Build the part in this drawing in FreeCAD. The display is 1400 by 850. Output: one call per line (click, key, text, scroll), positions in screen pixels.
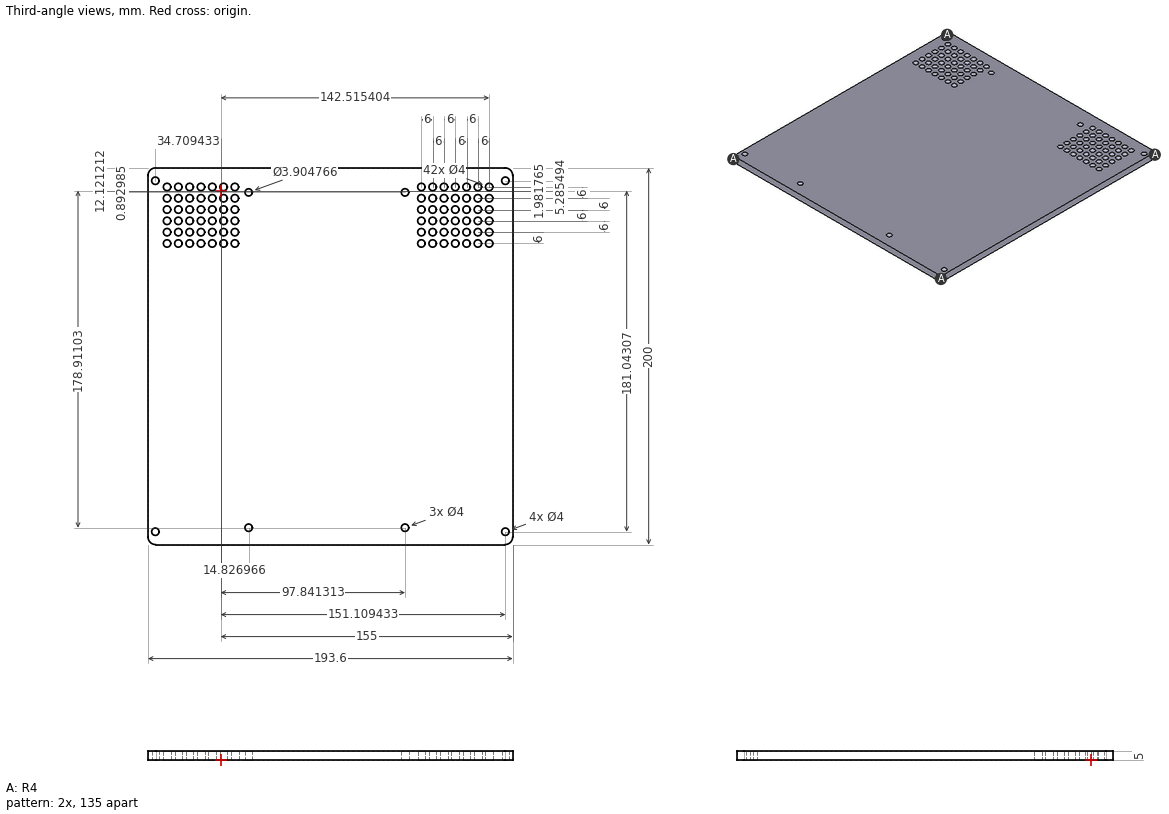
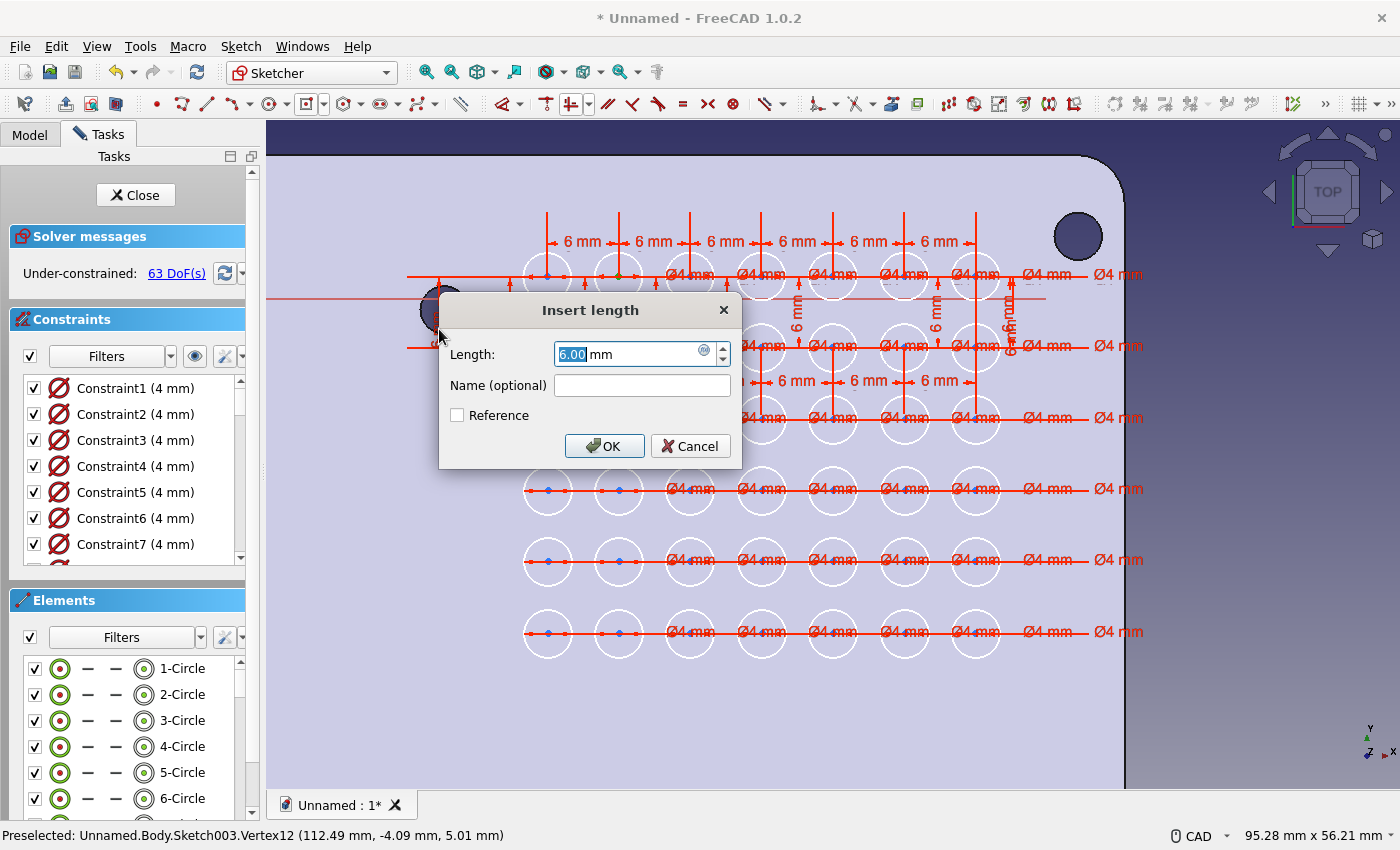
text(6)
key(Return)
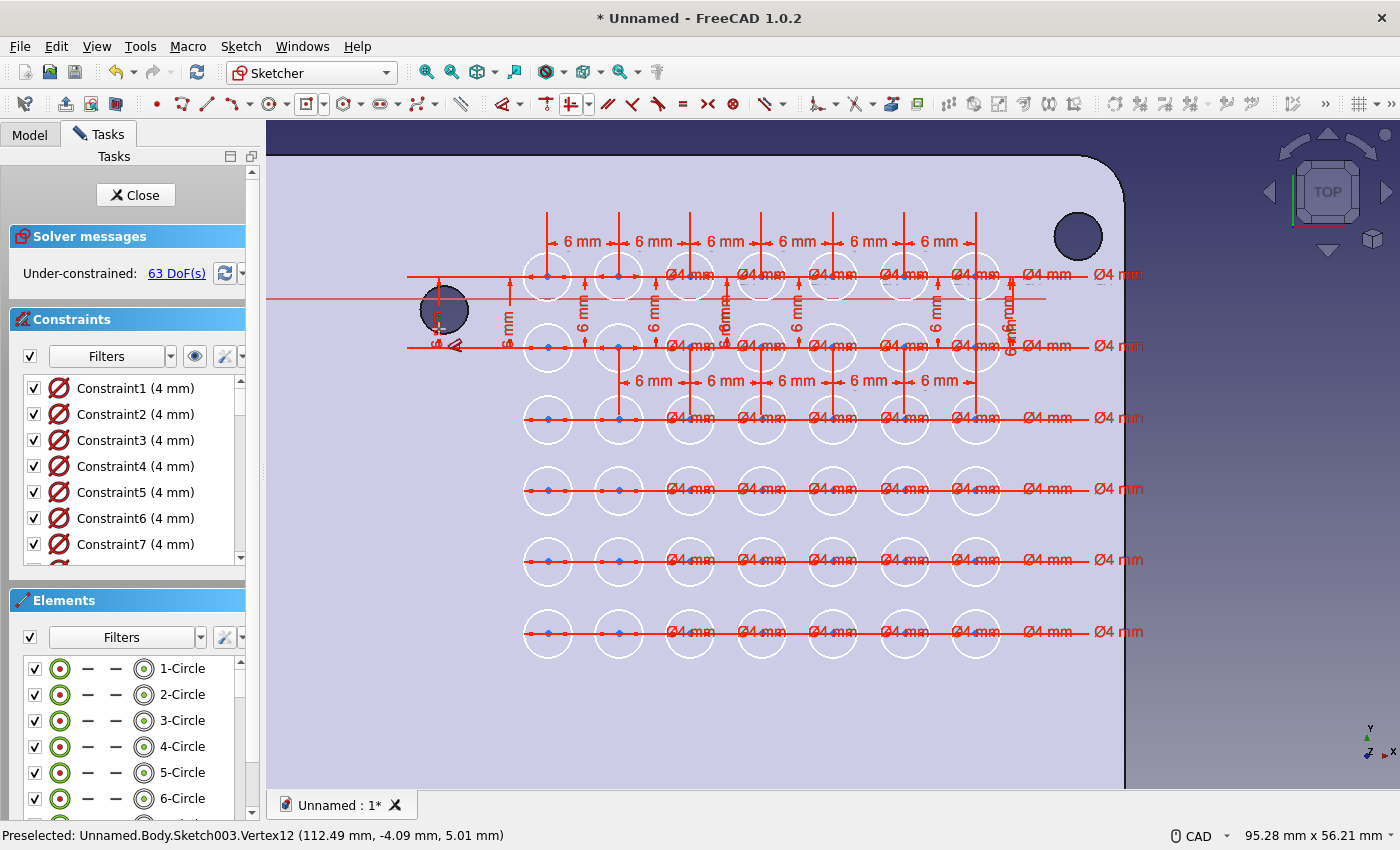
click(547, 277)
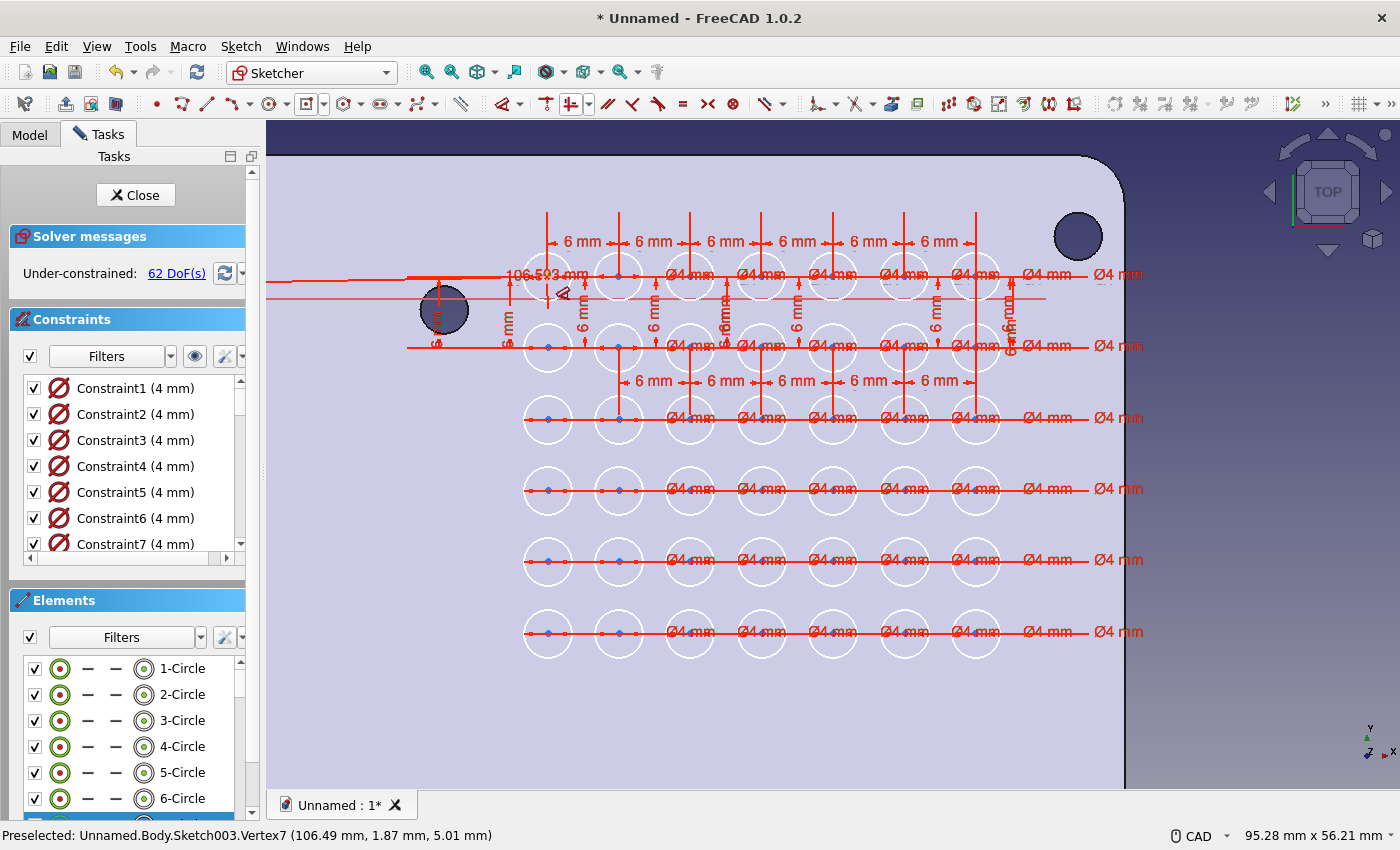
click(619, 348)
click(367, 313)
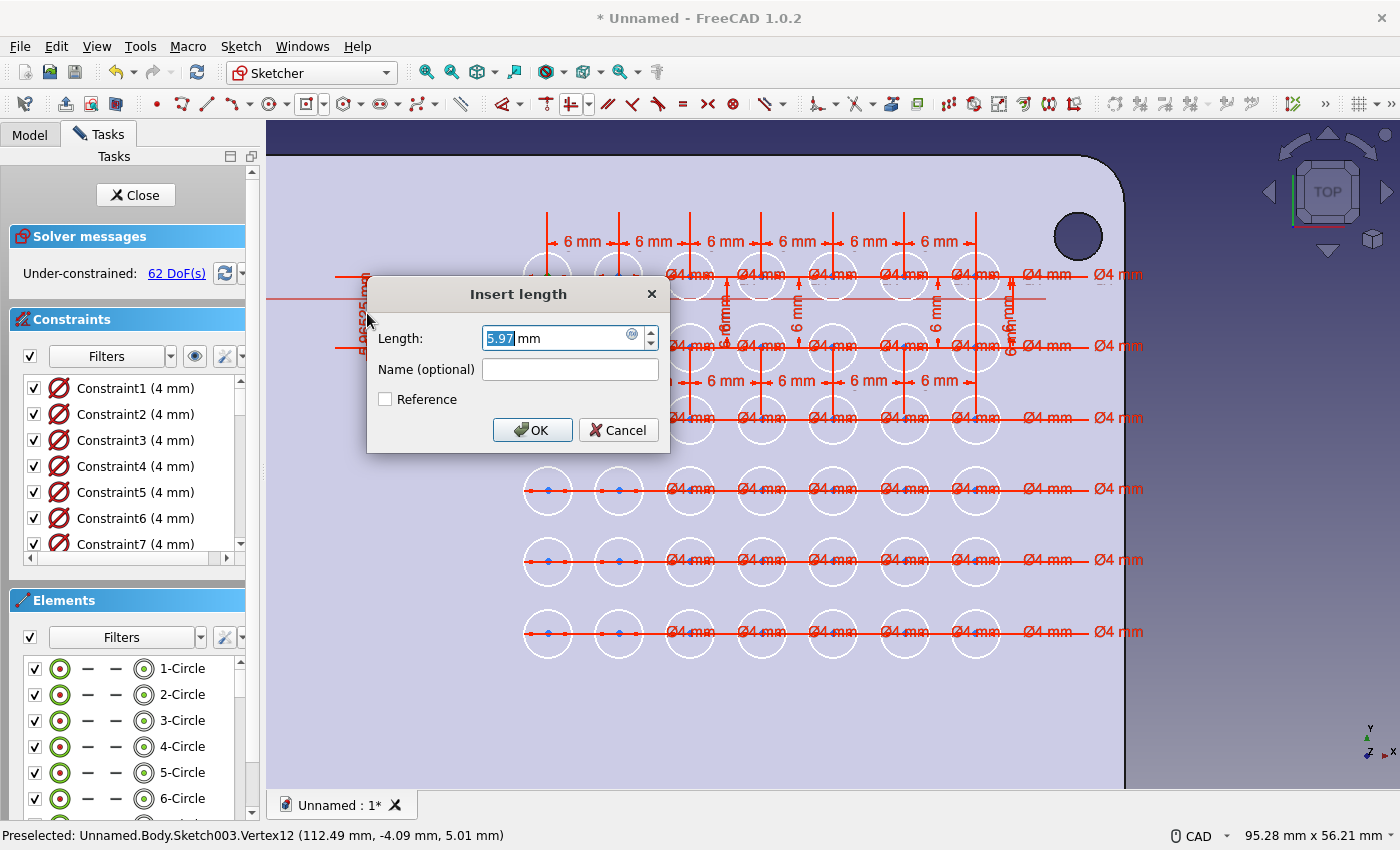
text(6)
key(Return)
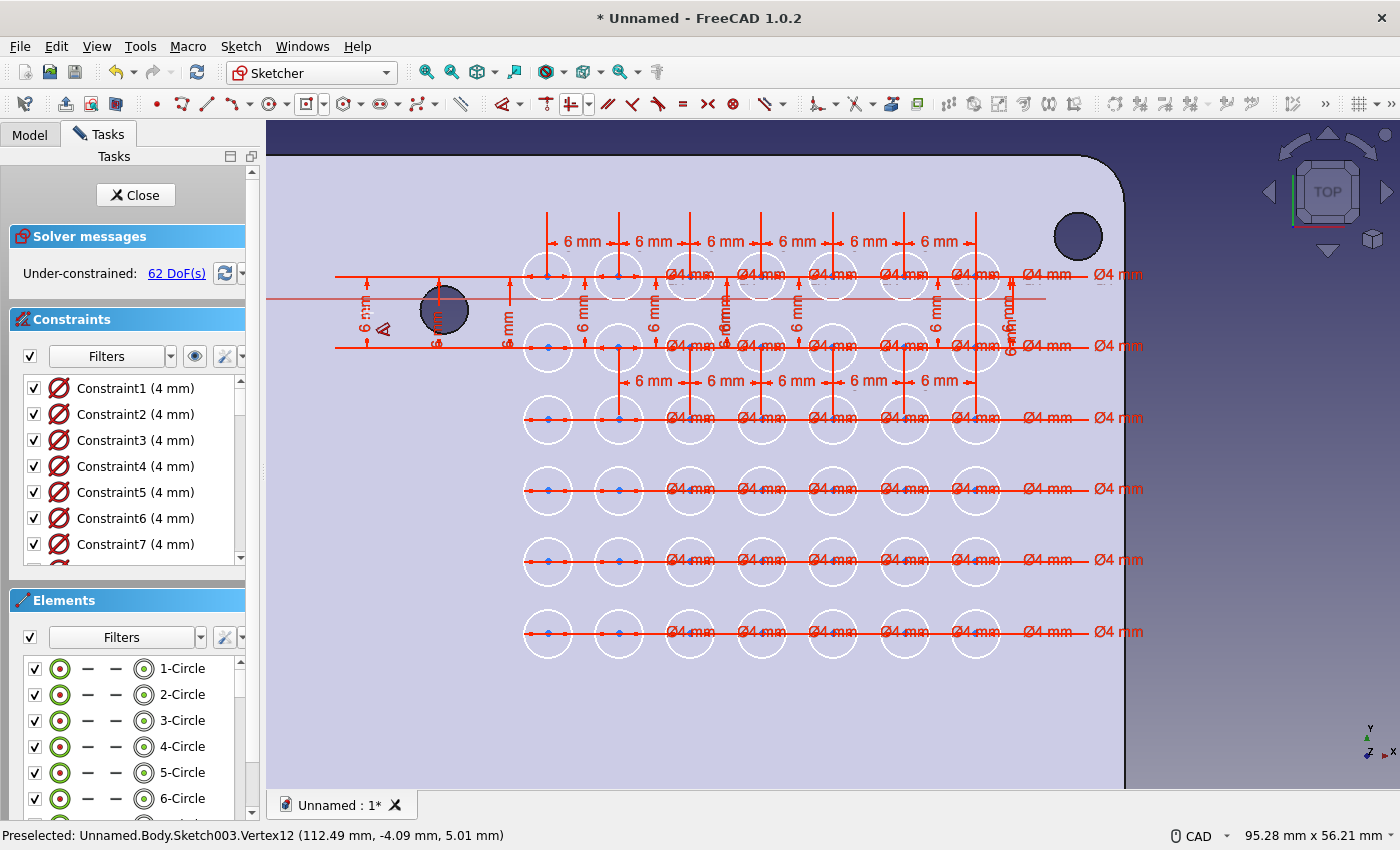
click(619, 348)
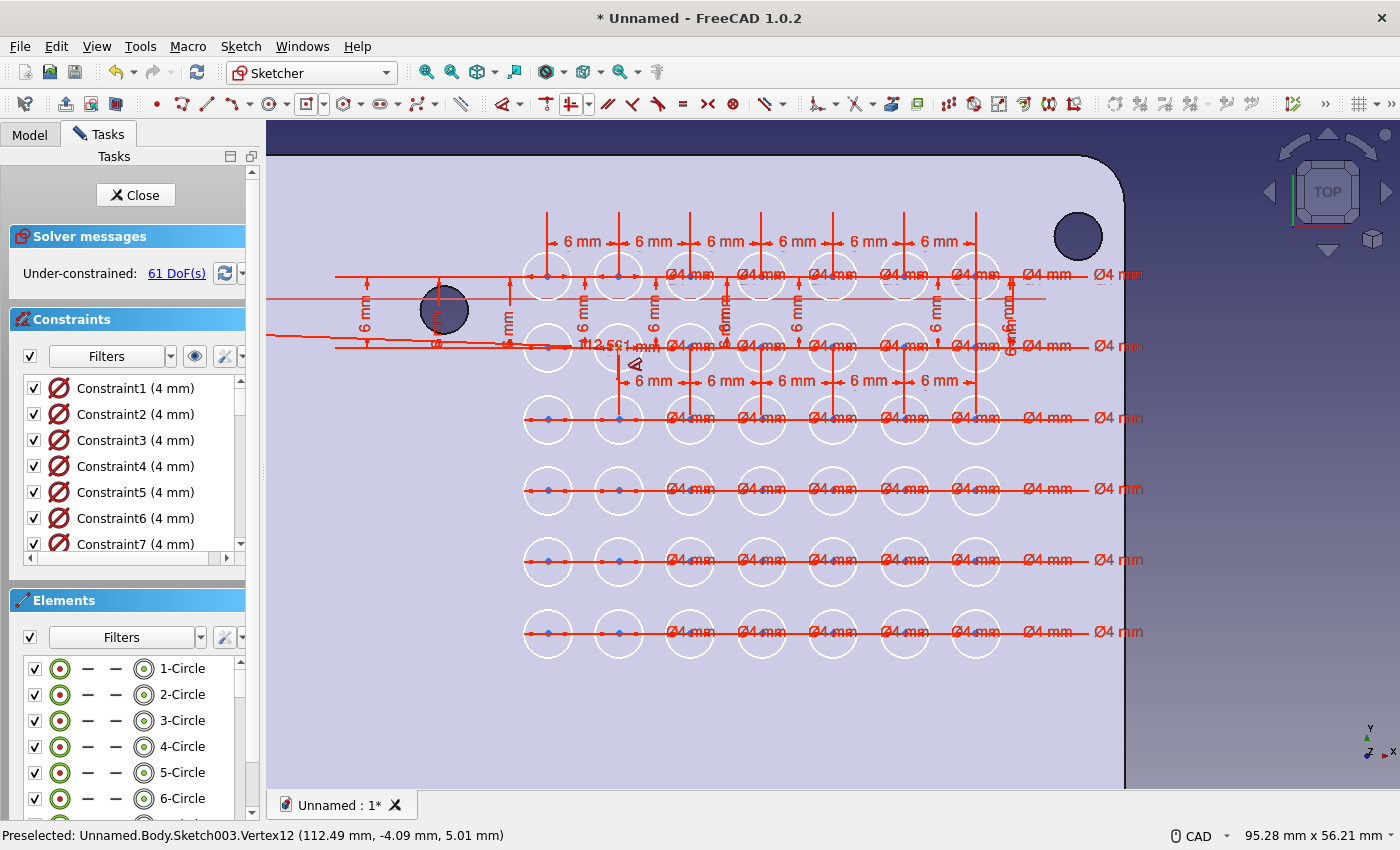
click(548, 348)
click(583, 382)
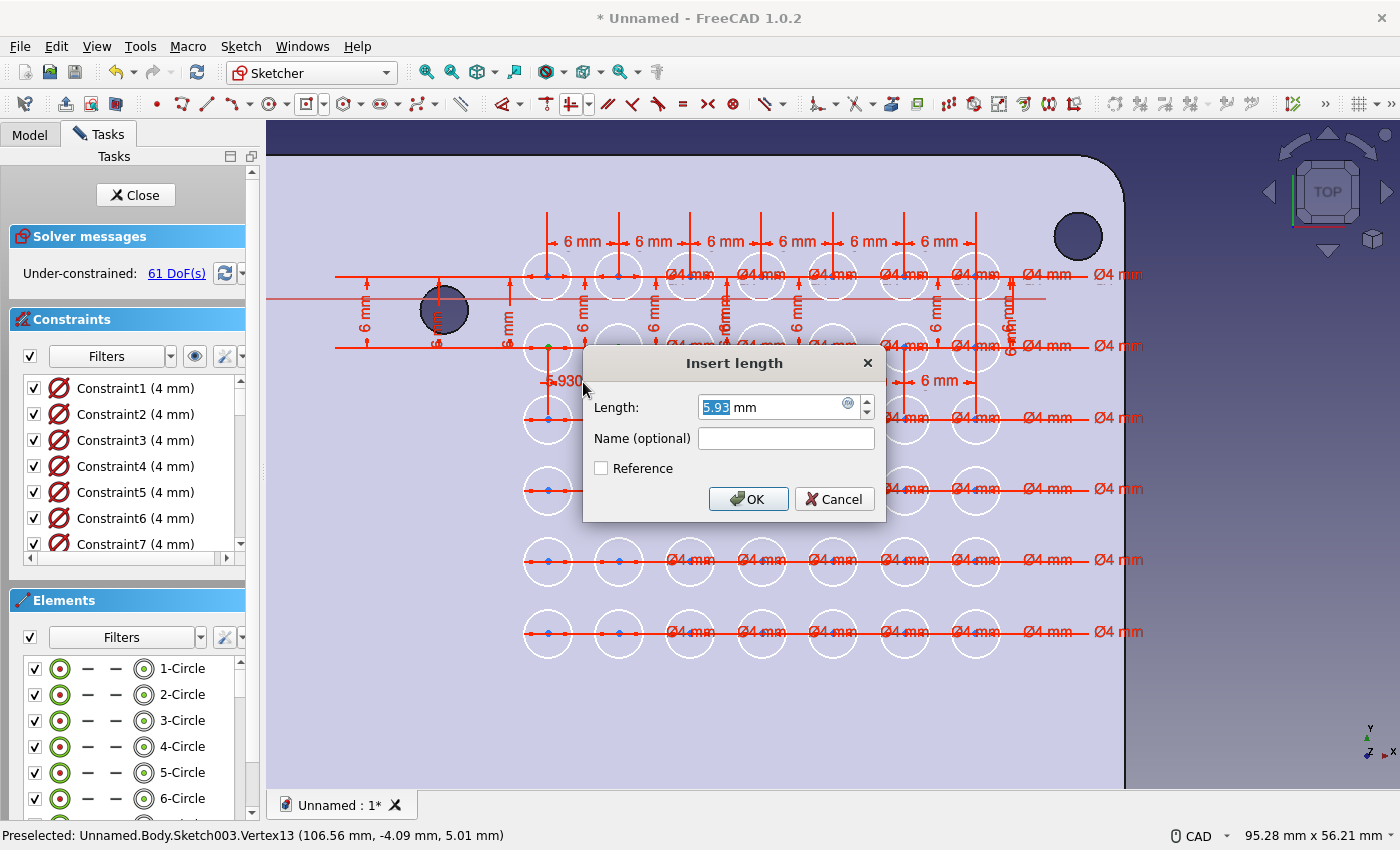
text(6)
key(Return)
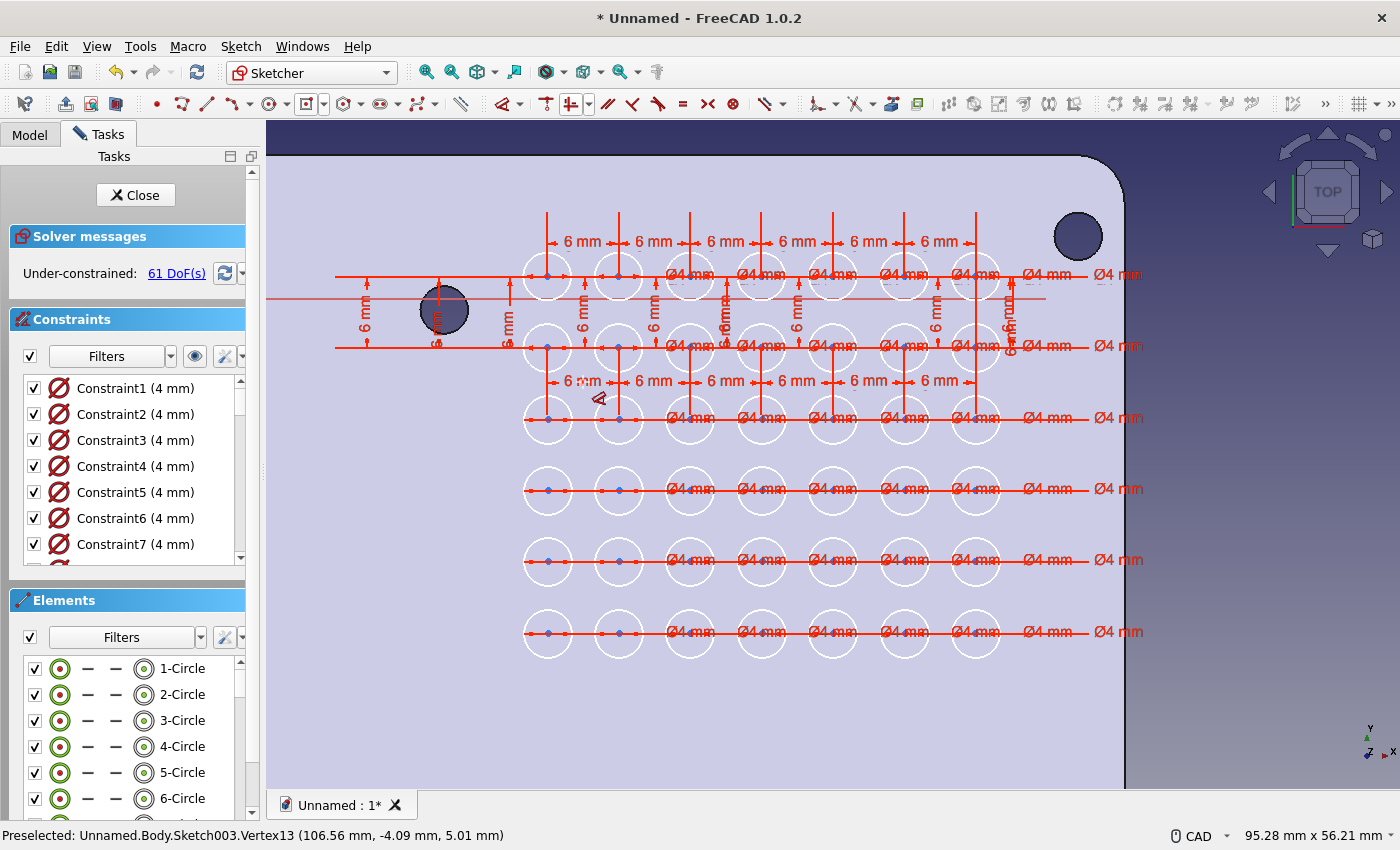
click(547, 277)